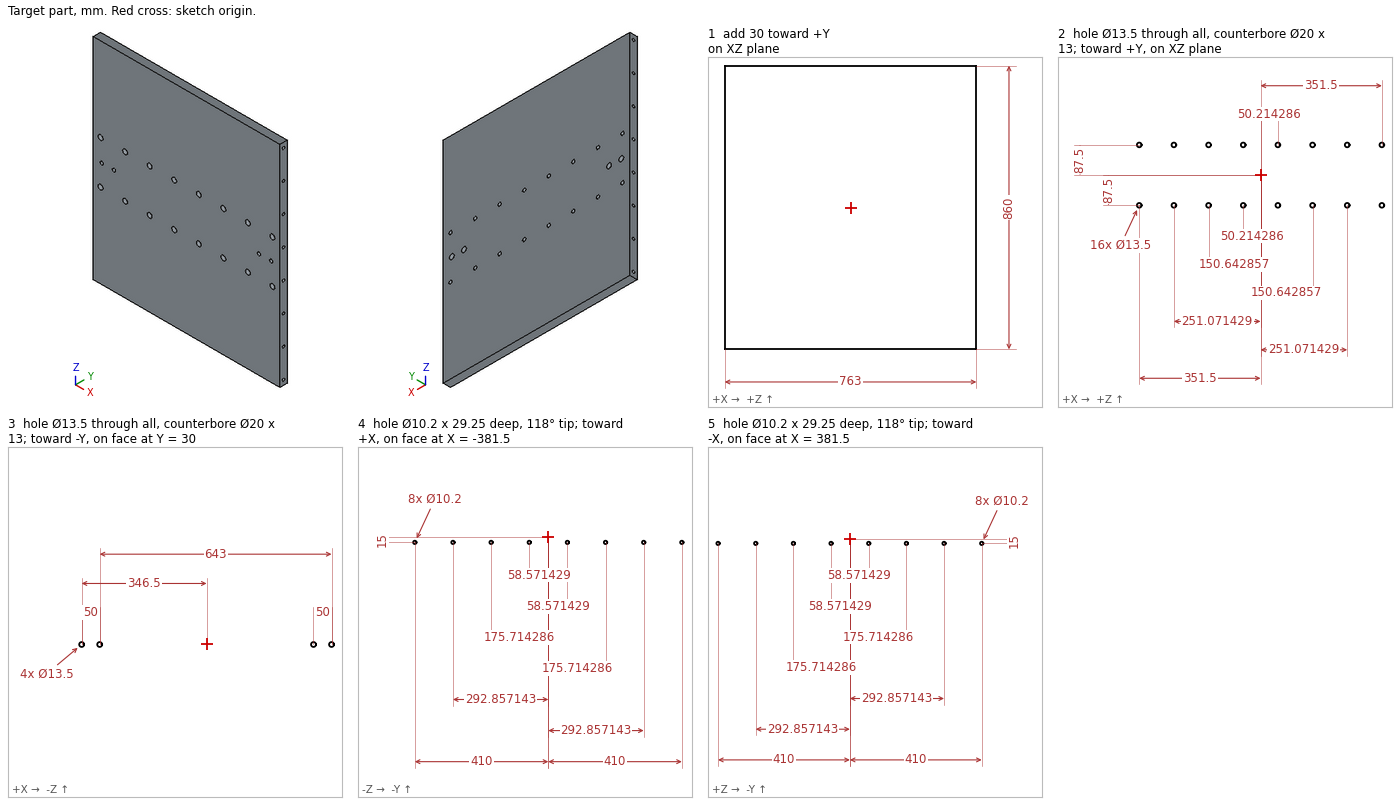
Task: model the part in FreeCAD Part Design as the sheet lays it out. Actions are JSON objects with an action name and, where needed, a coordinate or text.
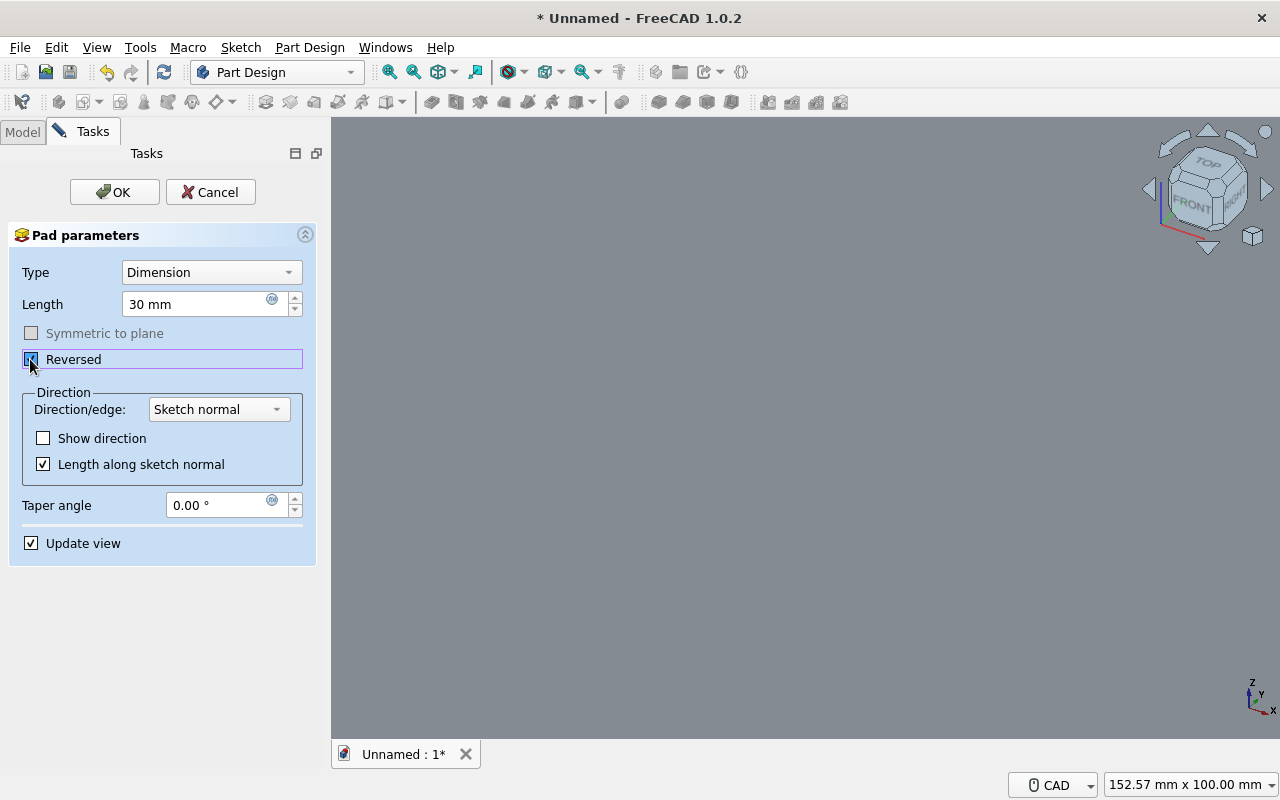
{"action": "left_click", "coordinate": [115, 192]}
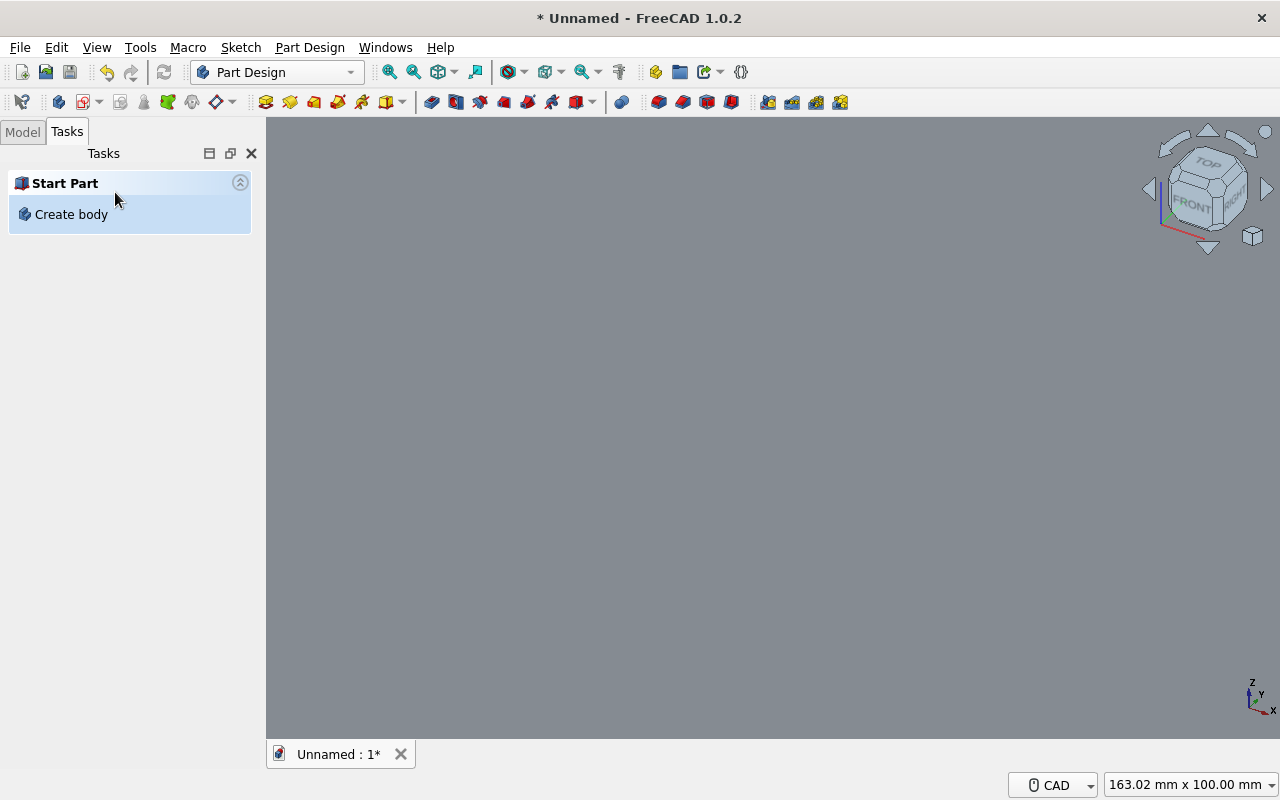
{"action": "left_click", "coordinate": [390, 72]}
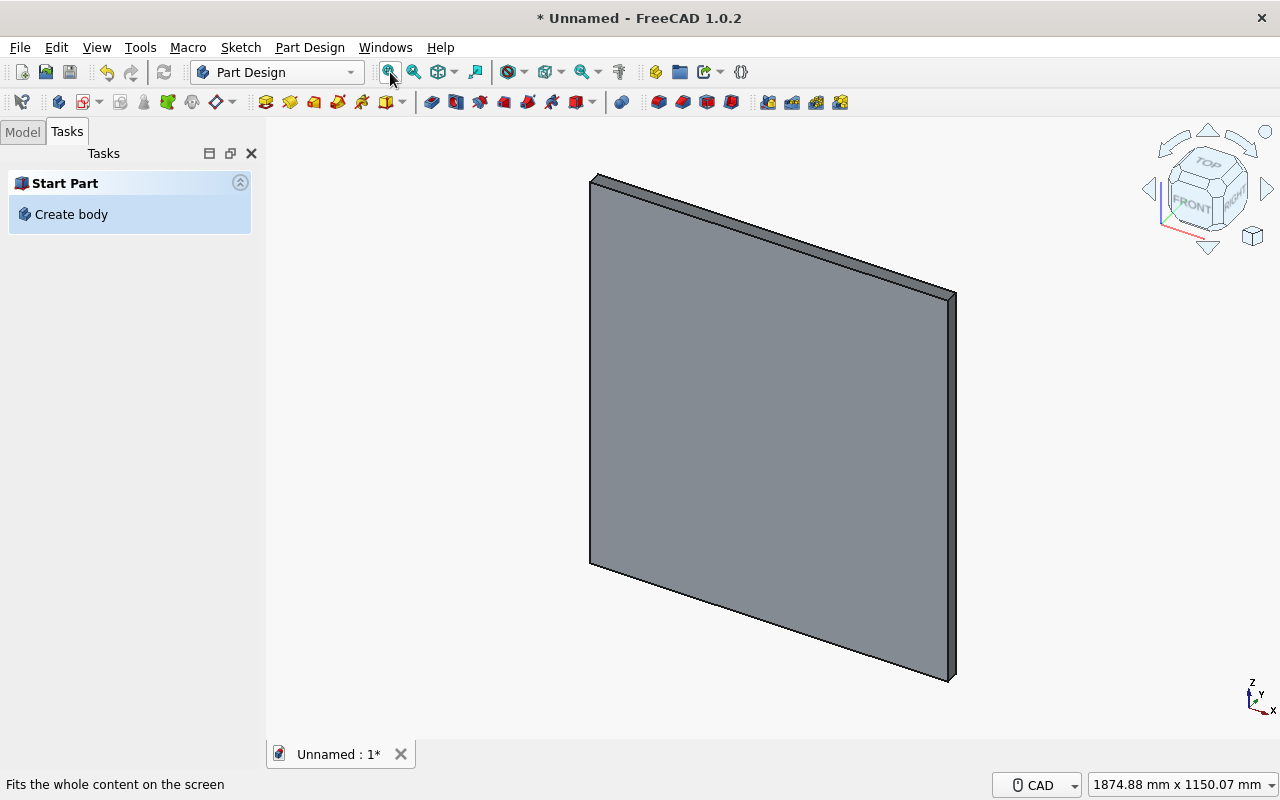
{"action": "left_click", "coordinate": [84, 102]}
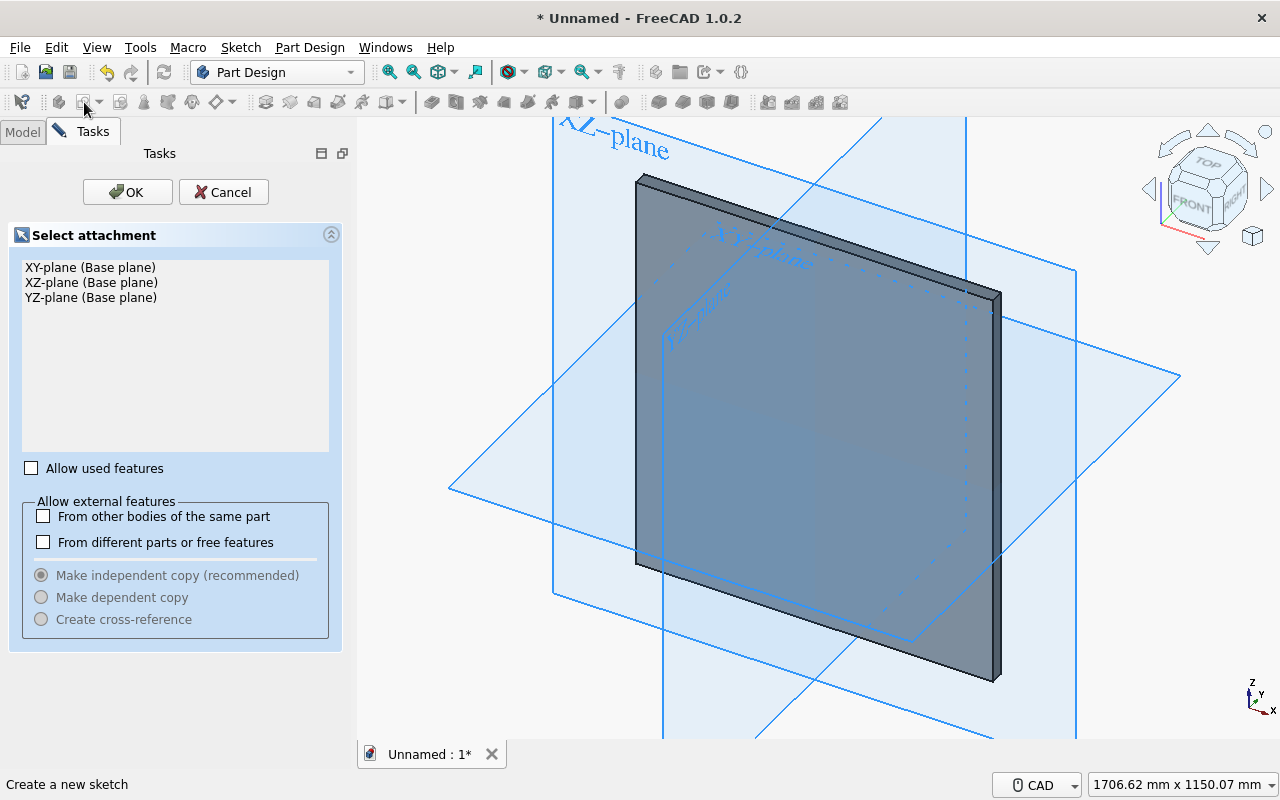
{"action": "left_click", "coordinate": [82, 282]}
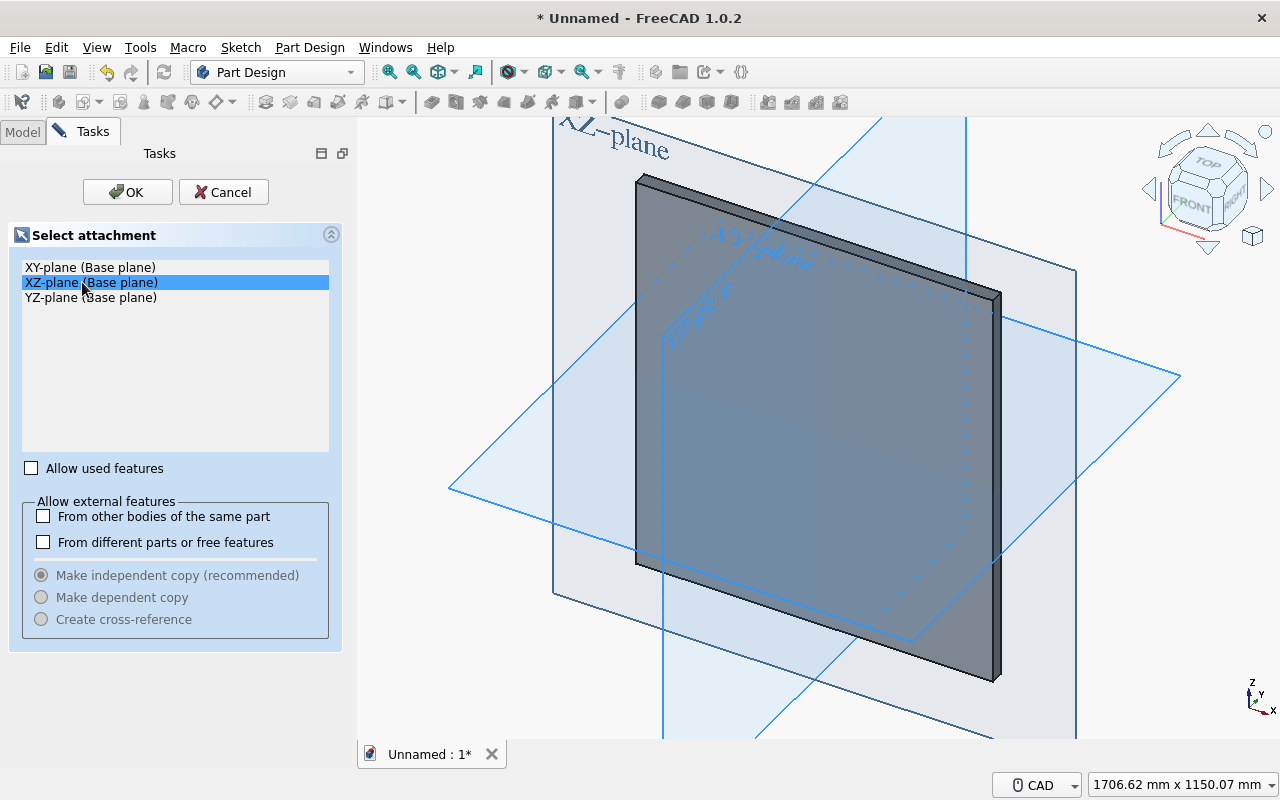
{"action": "left_click", "coordinate": [128, 192]}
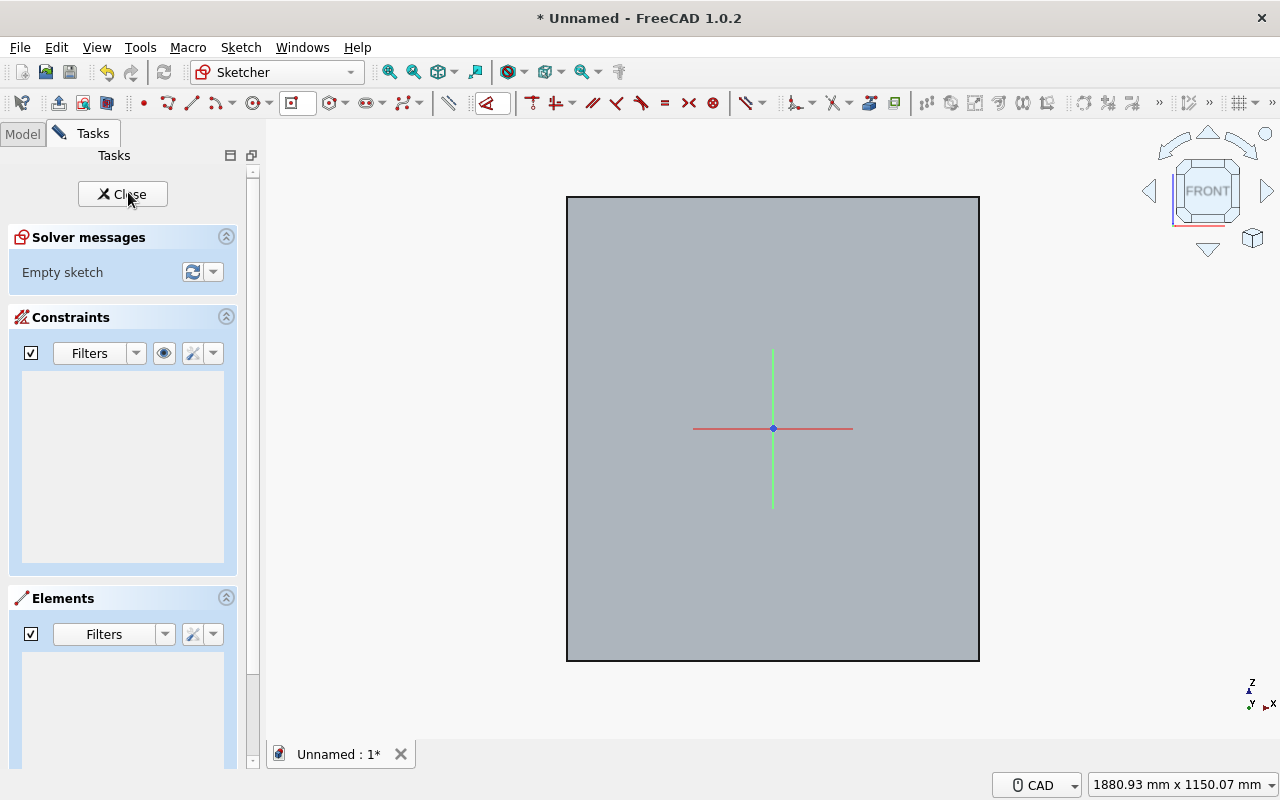
{"action": "scroll", "coordinate": [912, 429], "scroll_direction": "up", "scroll_amount": 2}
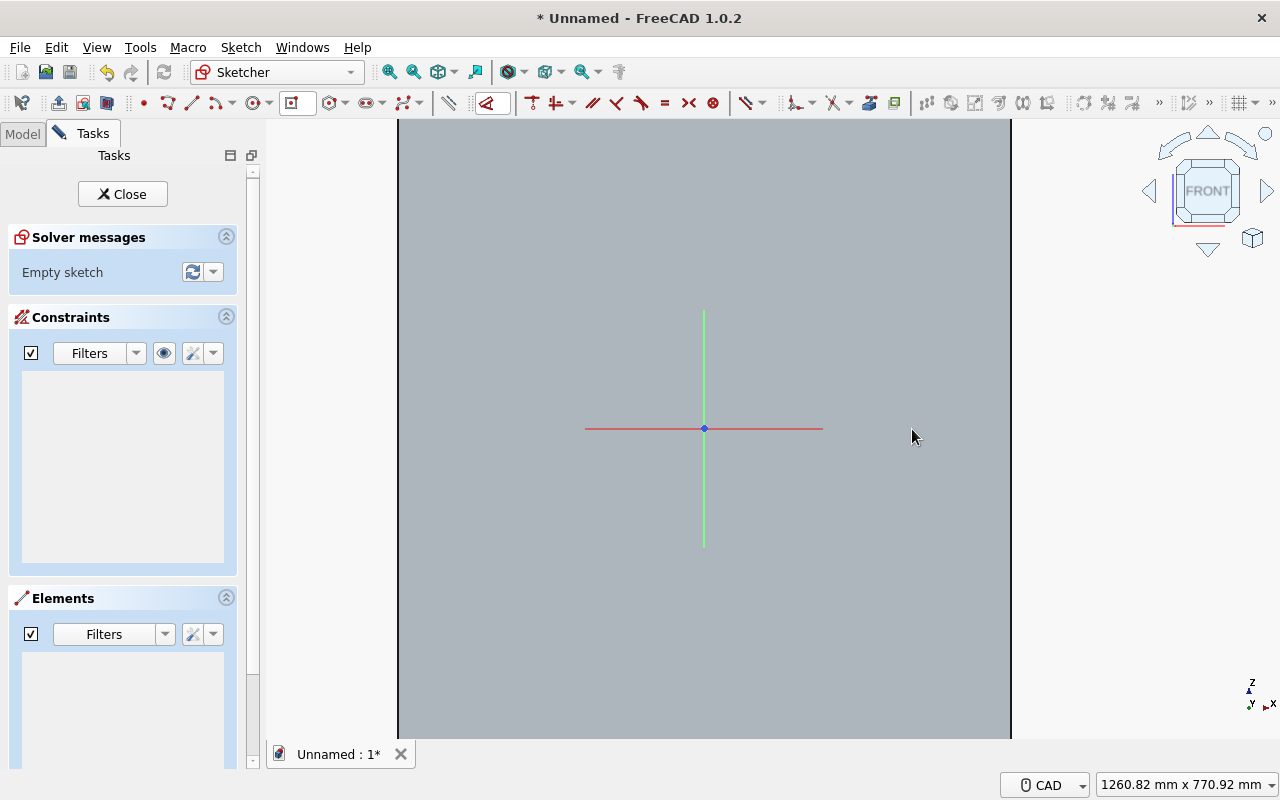
{"action": "left_click", "coordinate": [254, 104]}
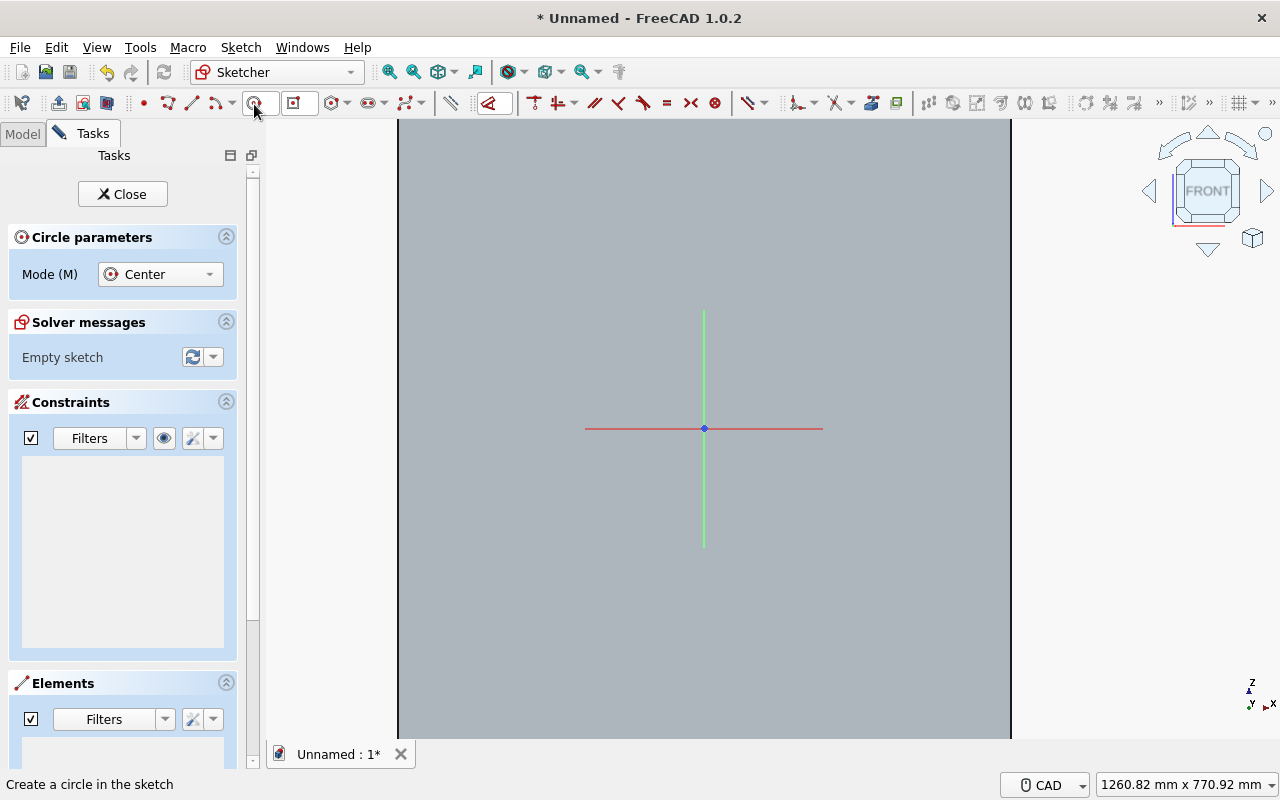
{"action": "scroll", "coordinate": [422, 499], "scroll_direction": "up", "scroll_amount": 8}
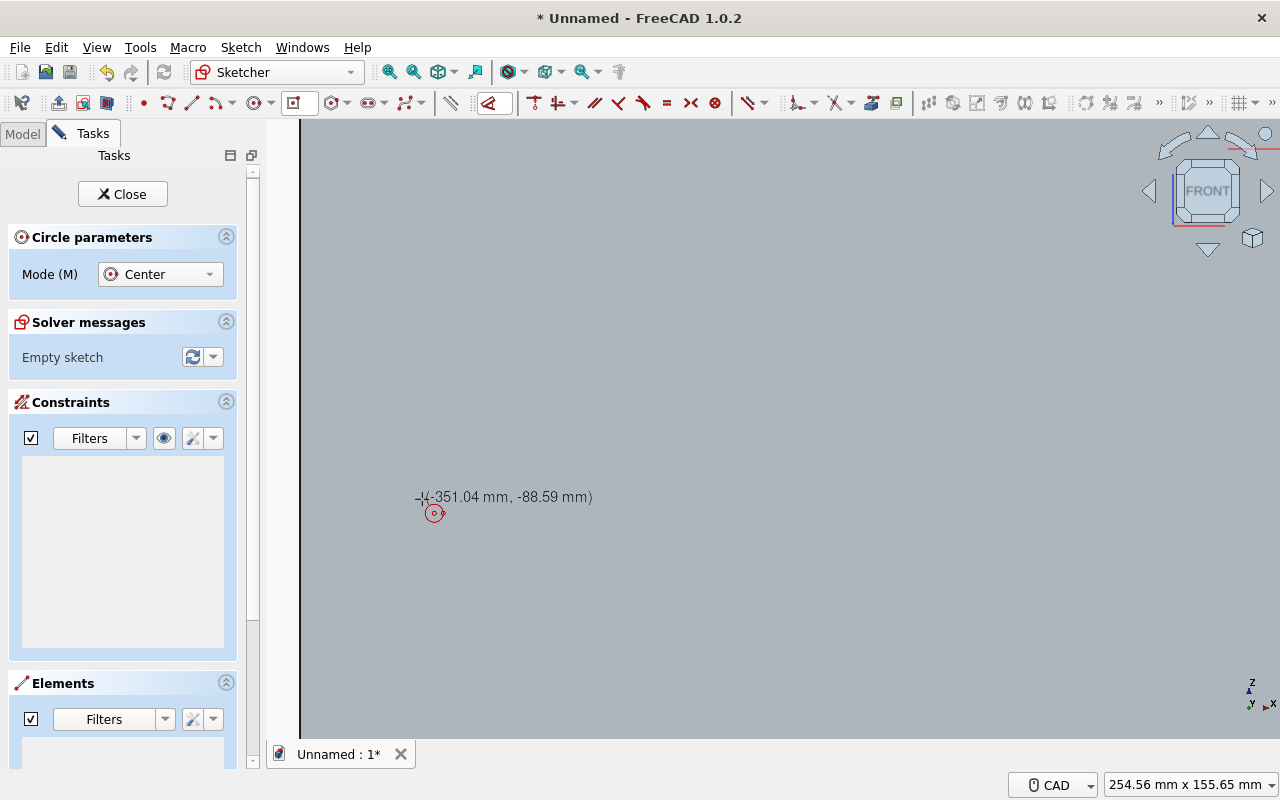
{"action": "scroll", "coordinate": [422, 500], "scroll_direction": "down", "scroll_amount": 8}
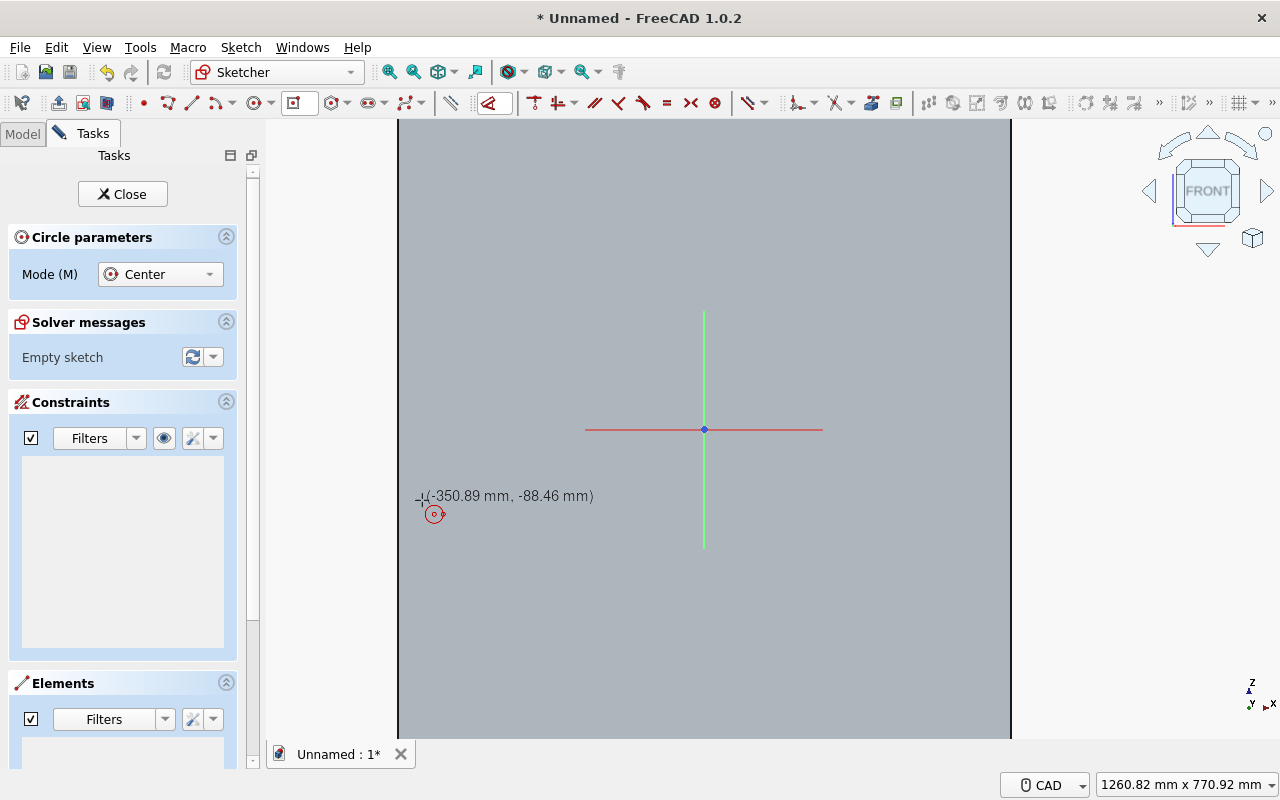
{"action": "left_click", "coordinate": [422, 500]}